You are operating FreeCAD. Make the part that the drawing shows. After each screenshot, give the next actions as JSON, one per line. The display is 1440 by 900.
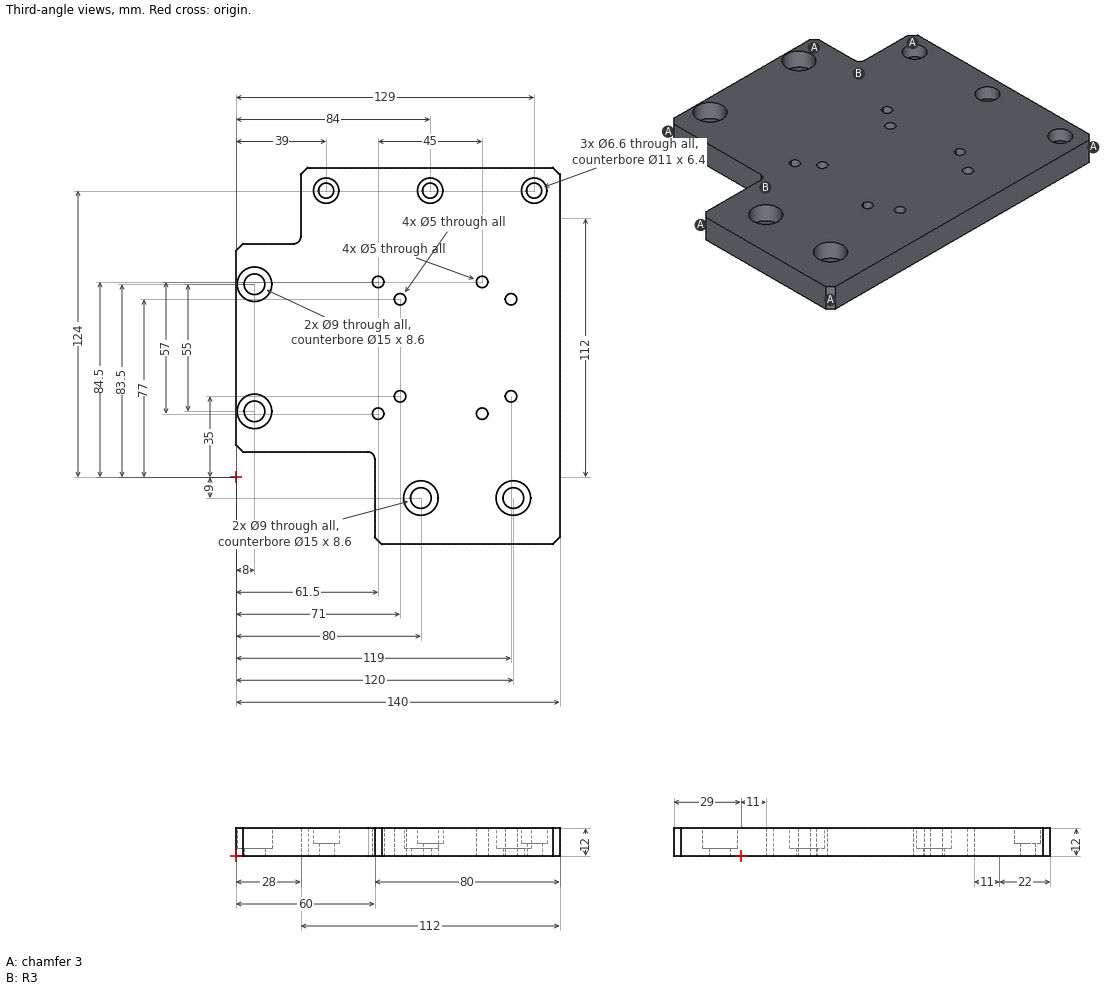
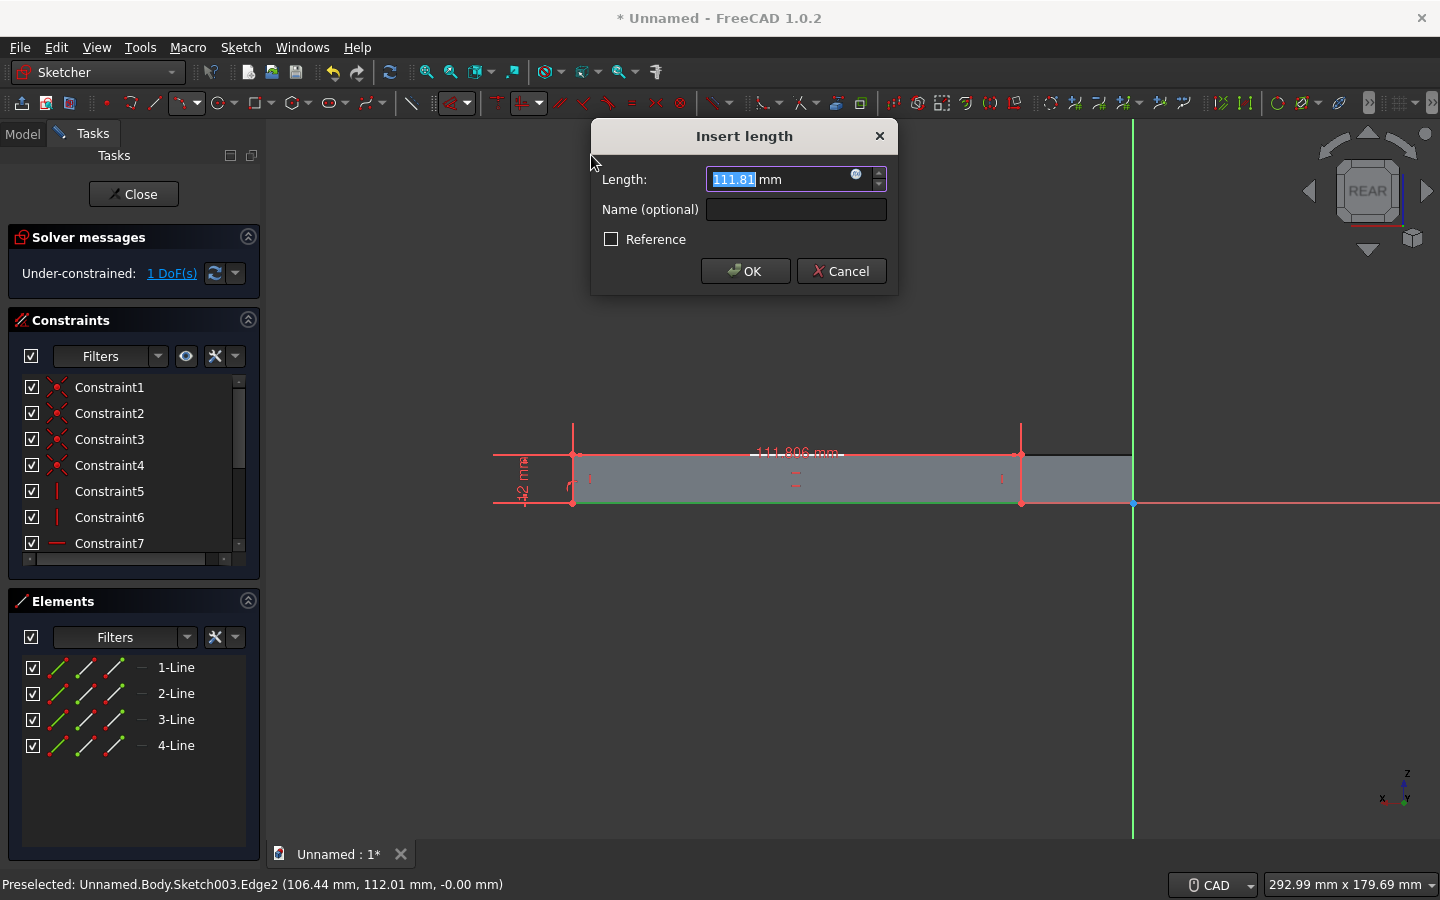
{"action": "type", "text": "112"}
{"action": "key", "text": "Return"}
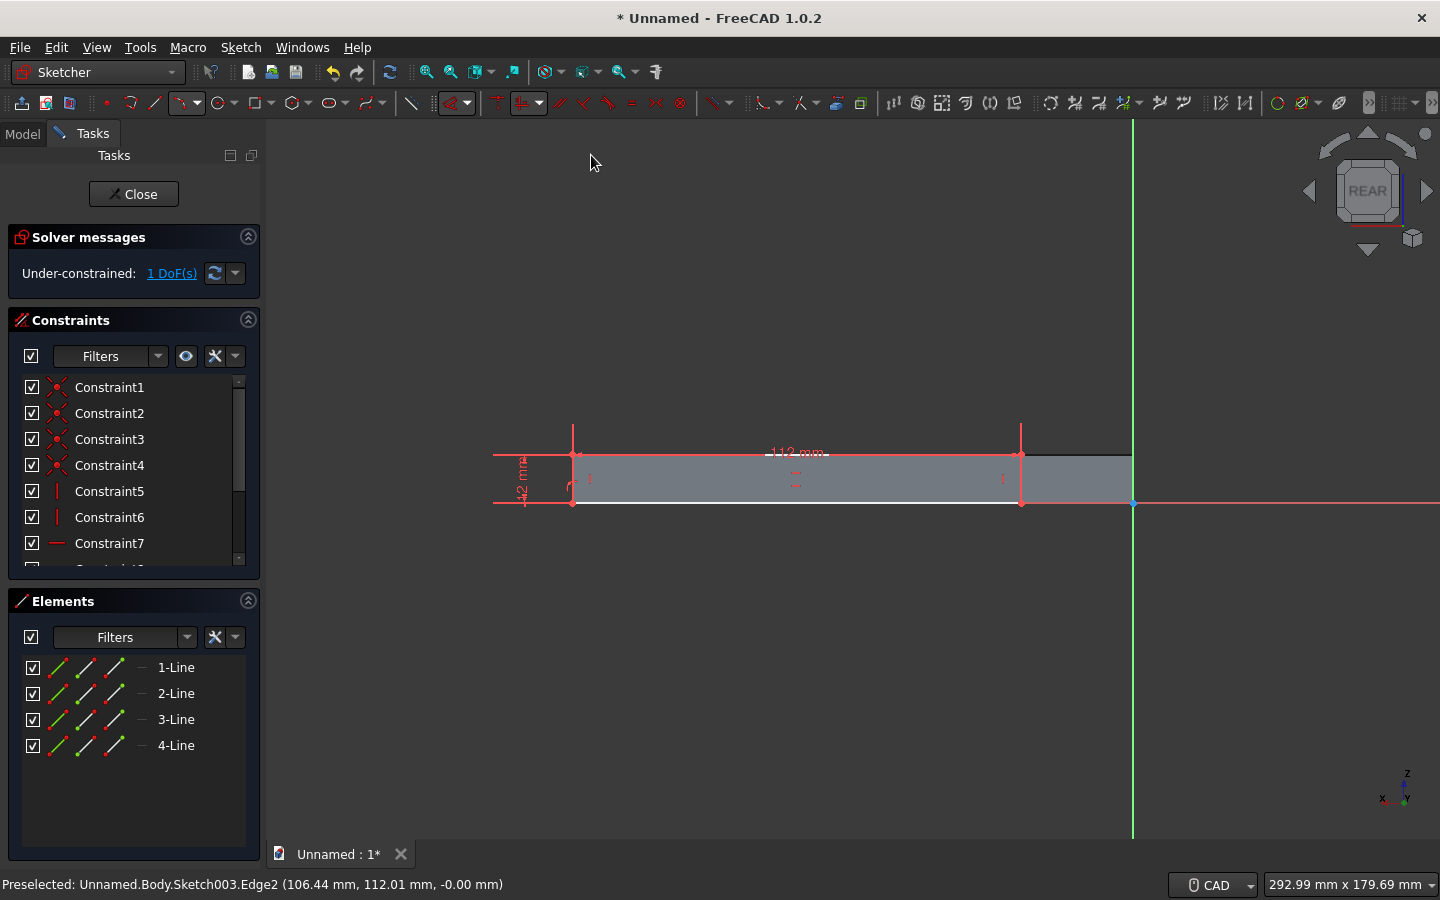
{"action": "left_click", "coordinate": [1021, 503]}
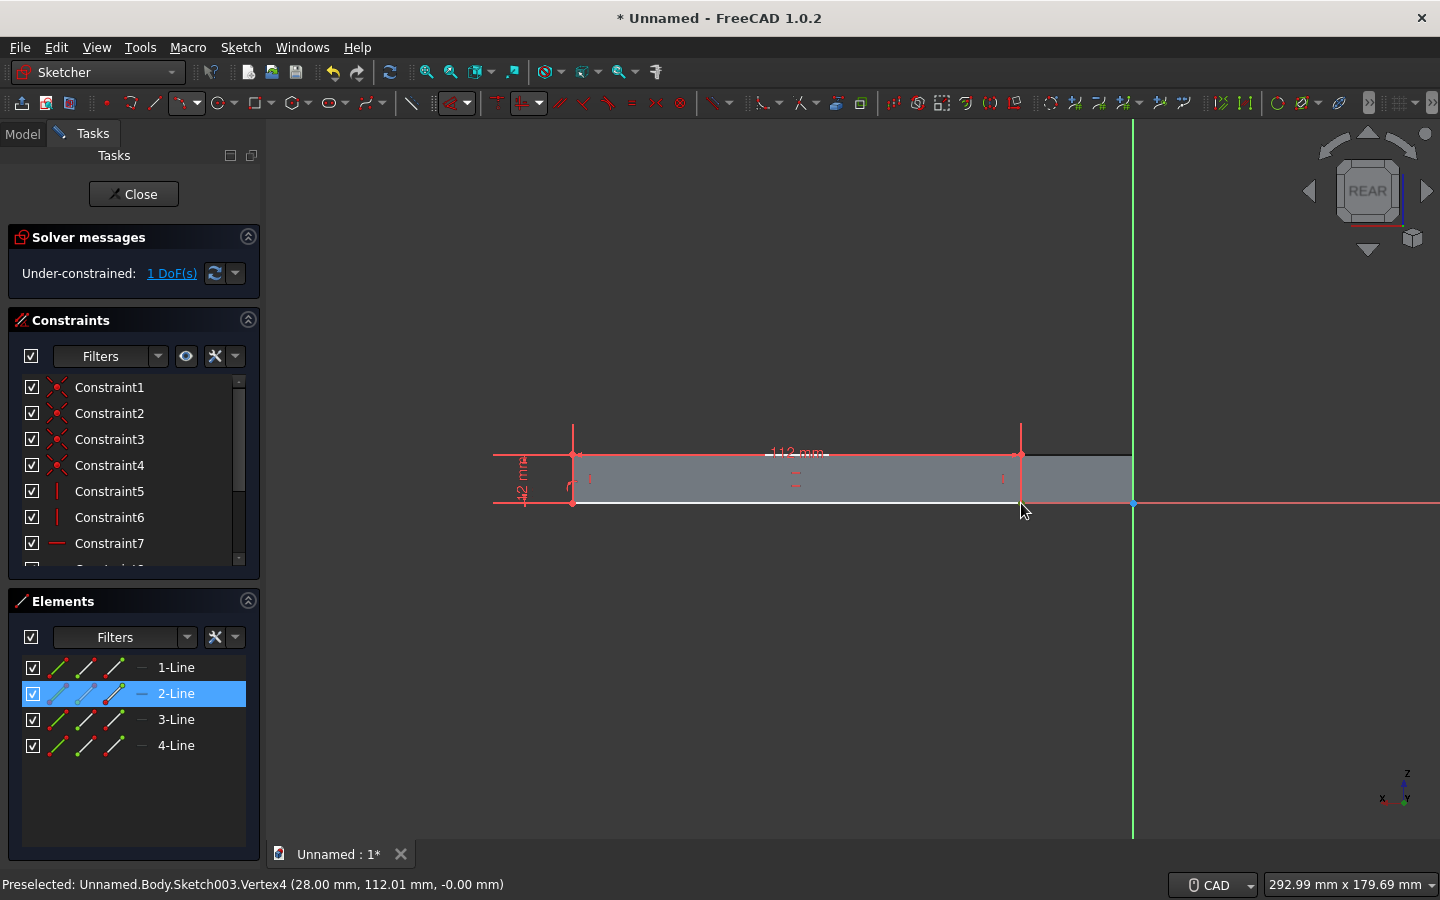
{"action": "left_click", "coordinate": [470, 104]}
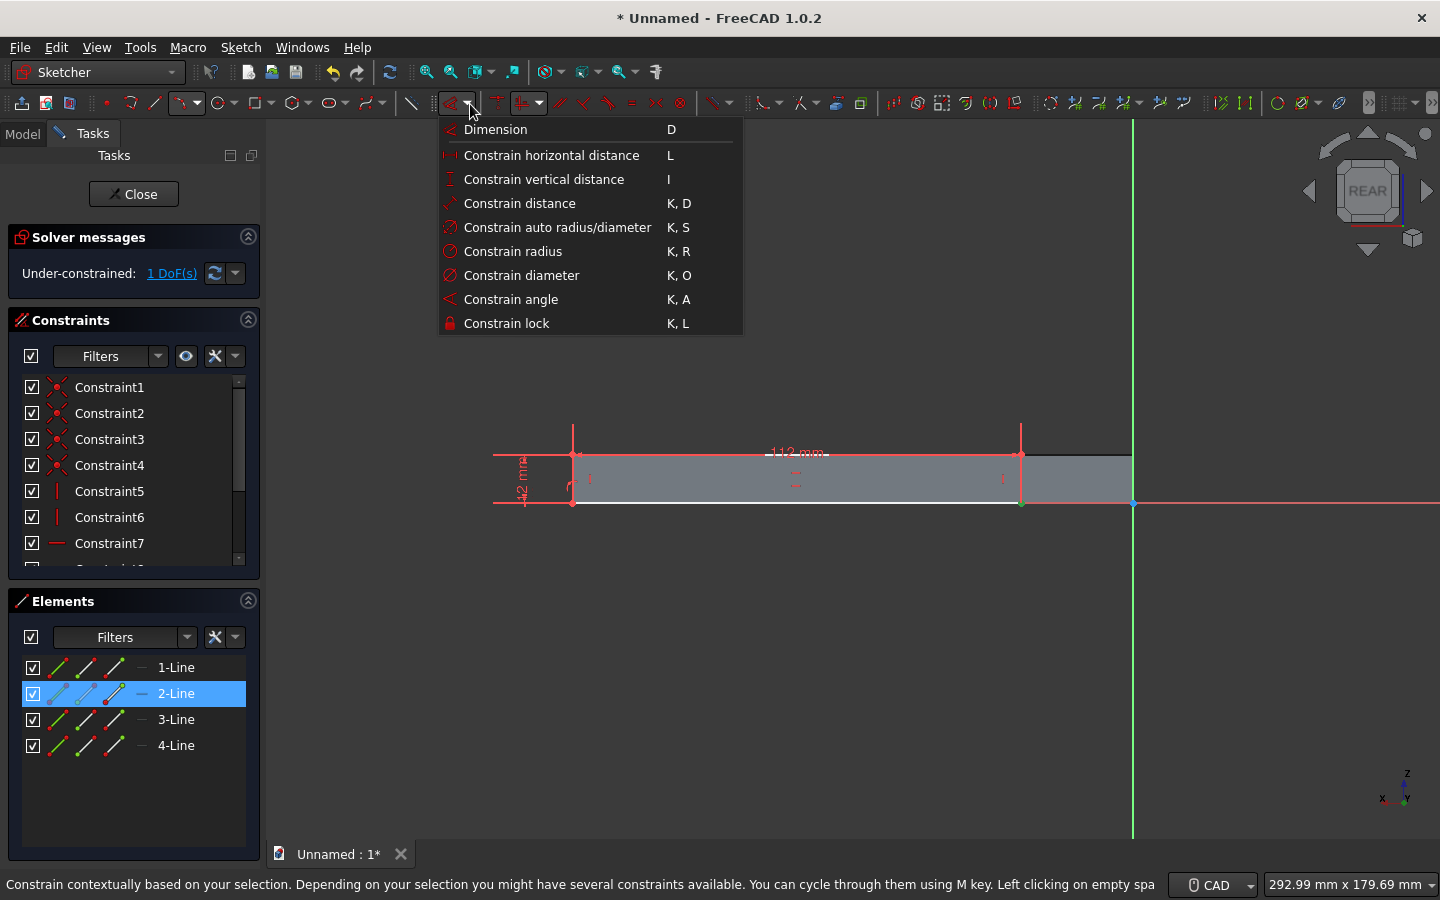
{"action": "left_click", "coordinate": [591, 155]}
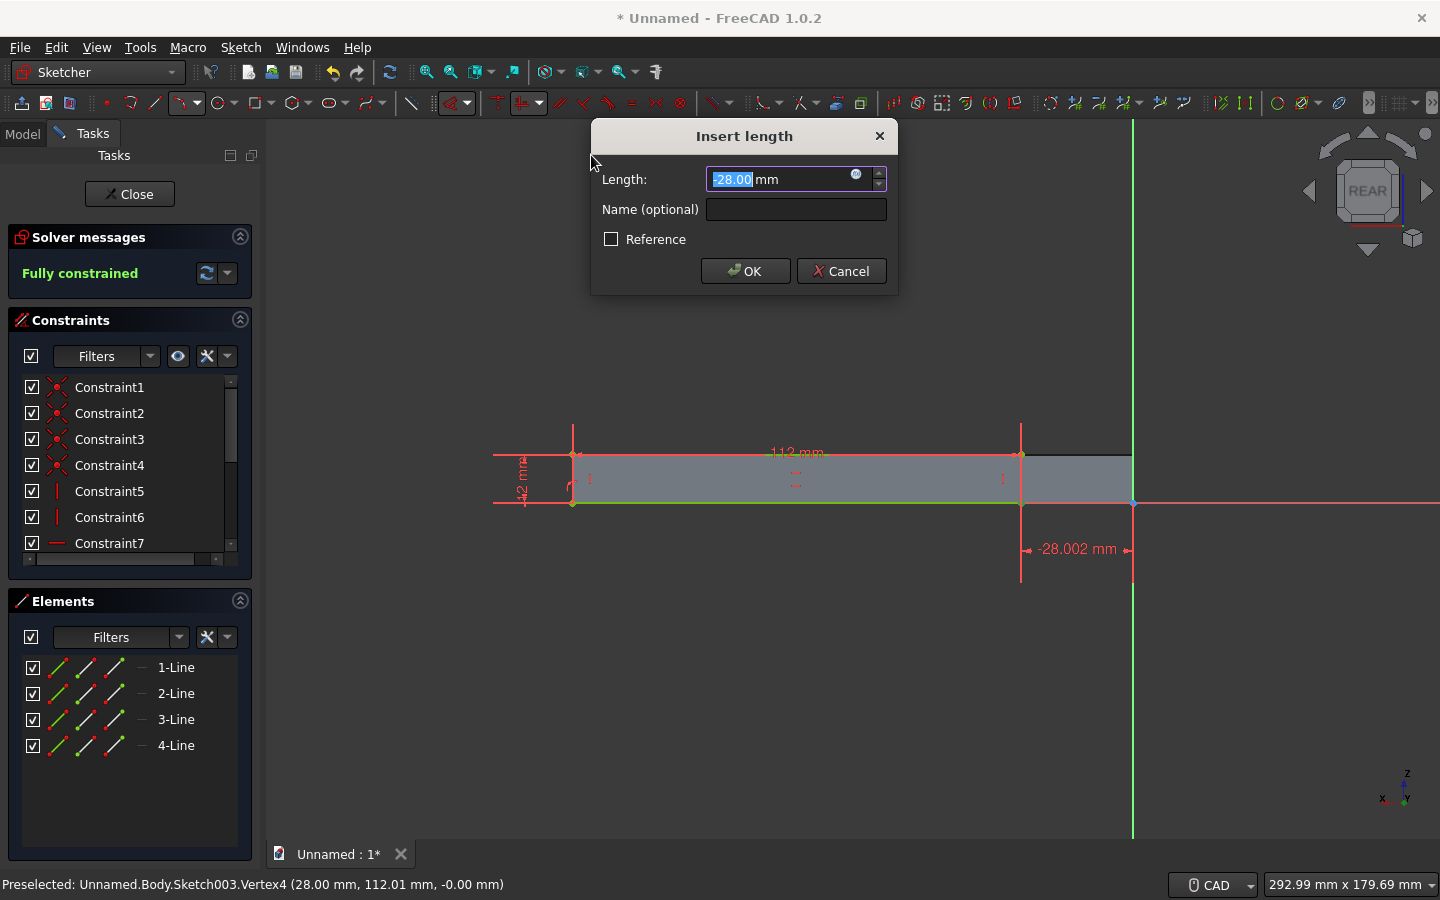
{"action": "type", "text": "-28"}
{"action": "key", "text": "Return"}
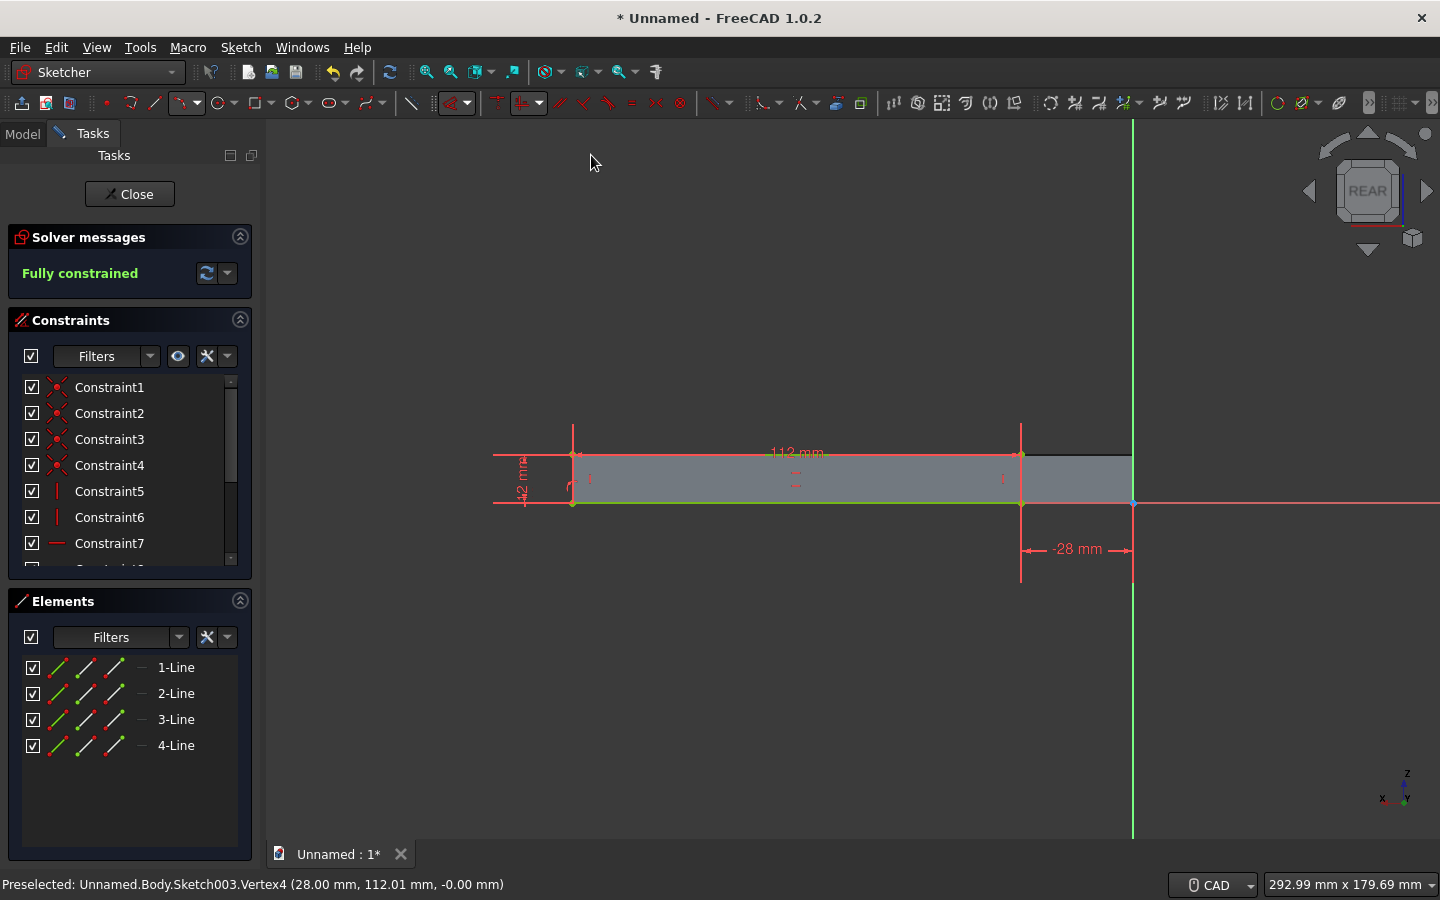
{"action": "left_click", "coordinate": [130, 194]}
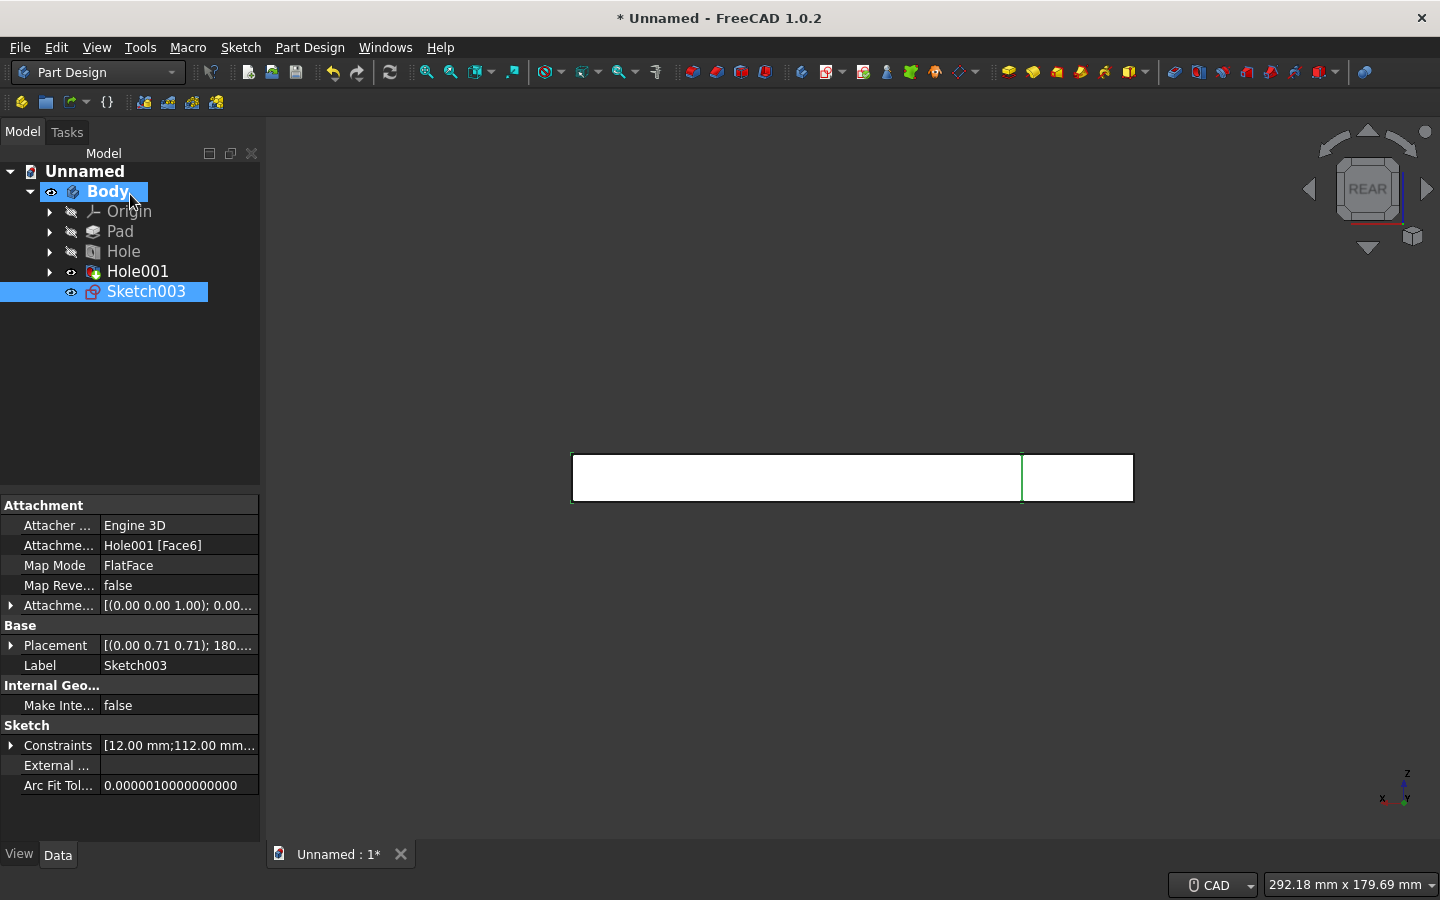
{"action": "left_click", "coordinate": [1010, 72]}